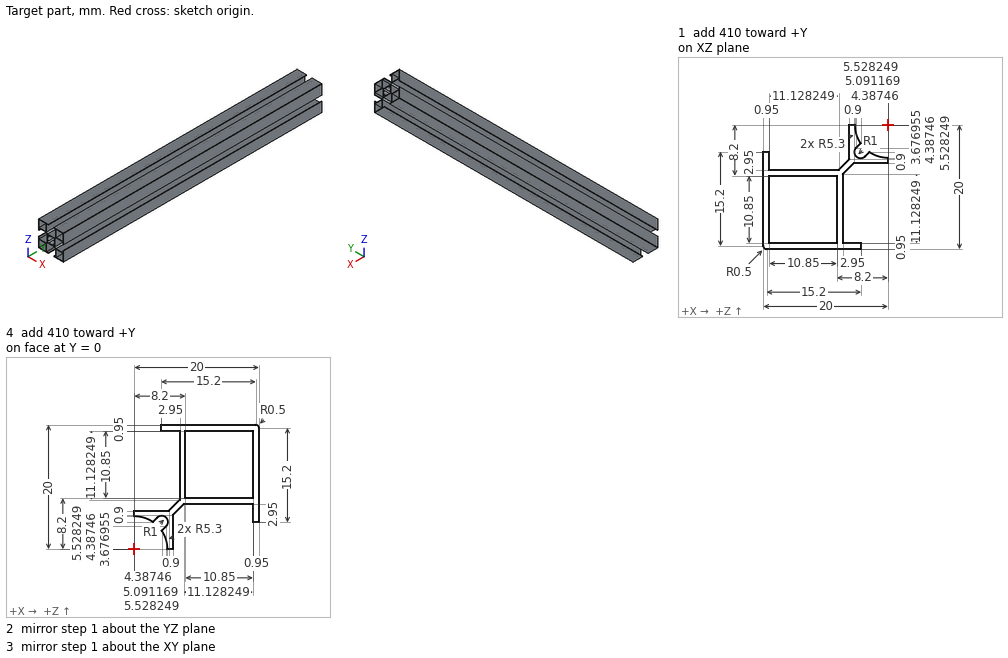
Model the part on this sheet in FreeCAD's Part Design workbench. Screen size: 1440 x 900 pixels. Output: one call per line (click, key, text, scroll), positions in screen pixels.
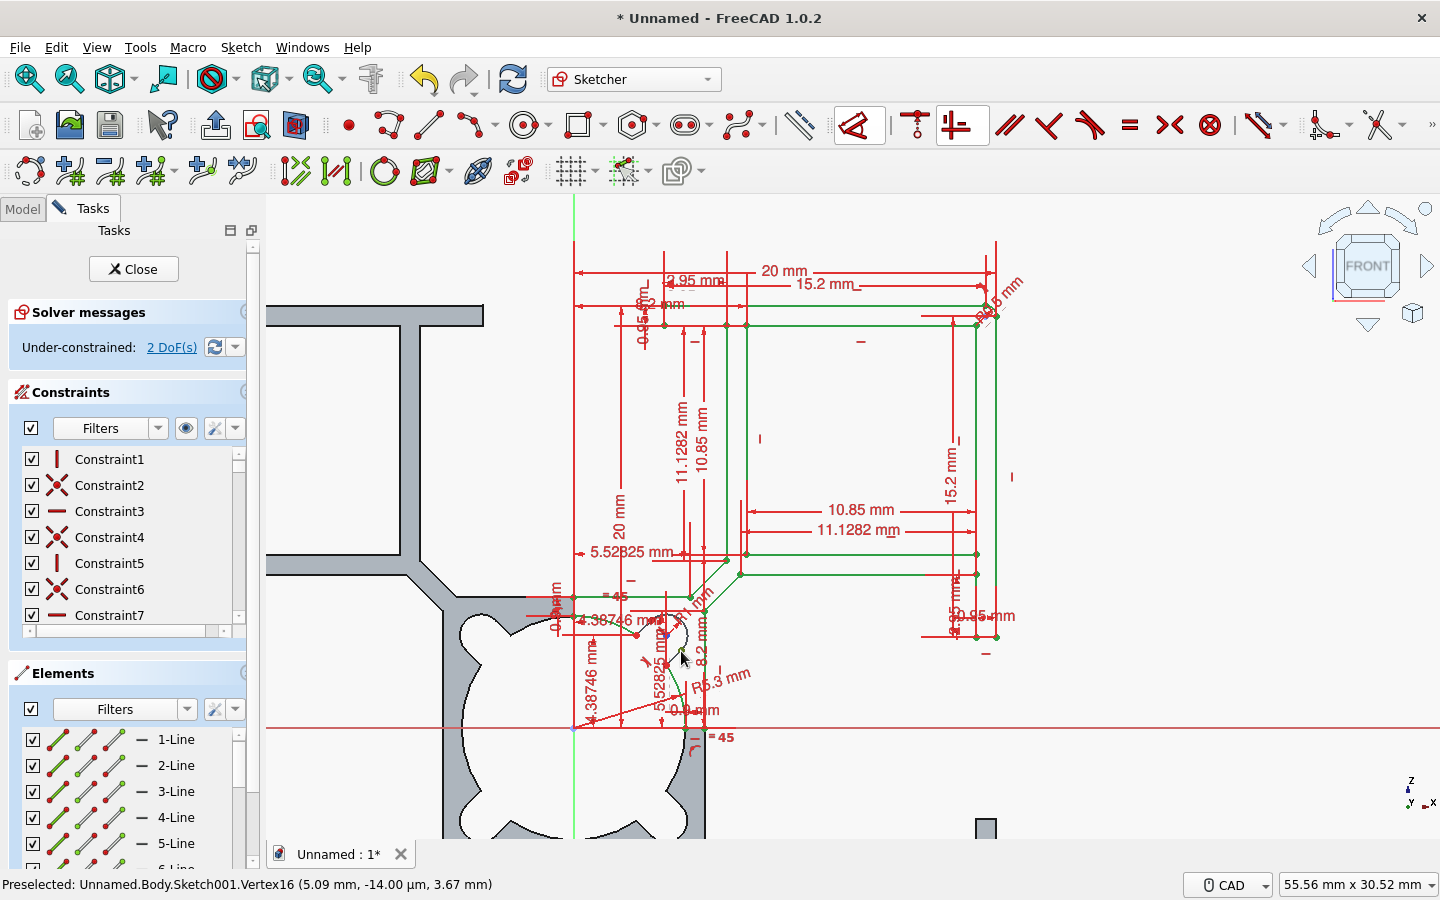
key(l)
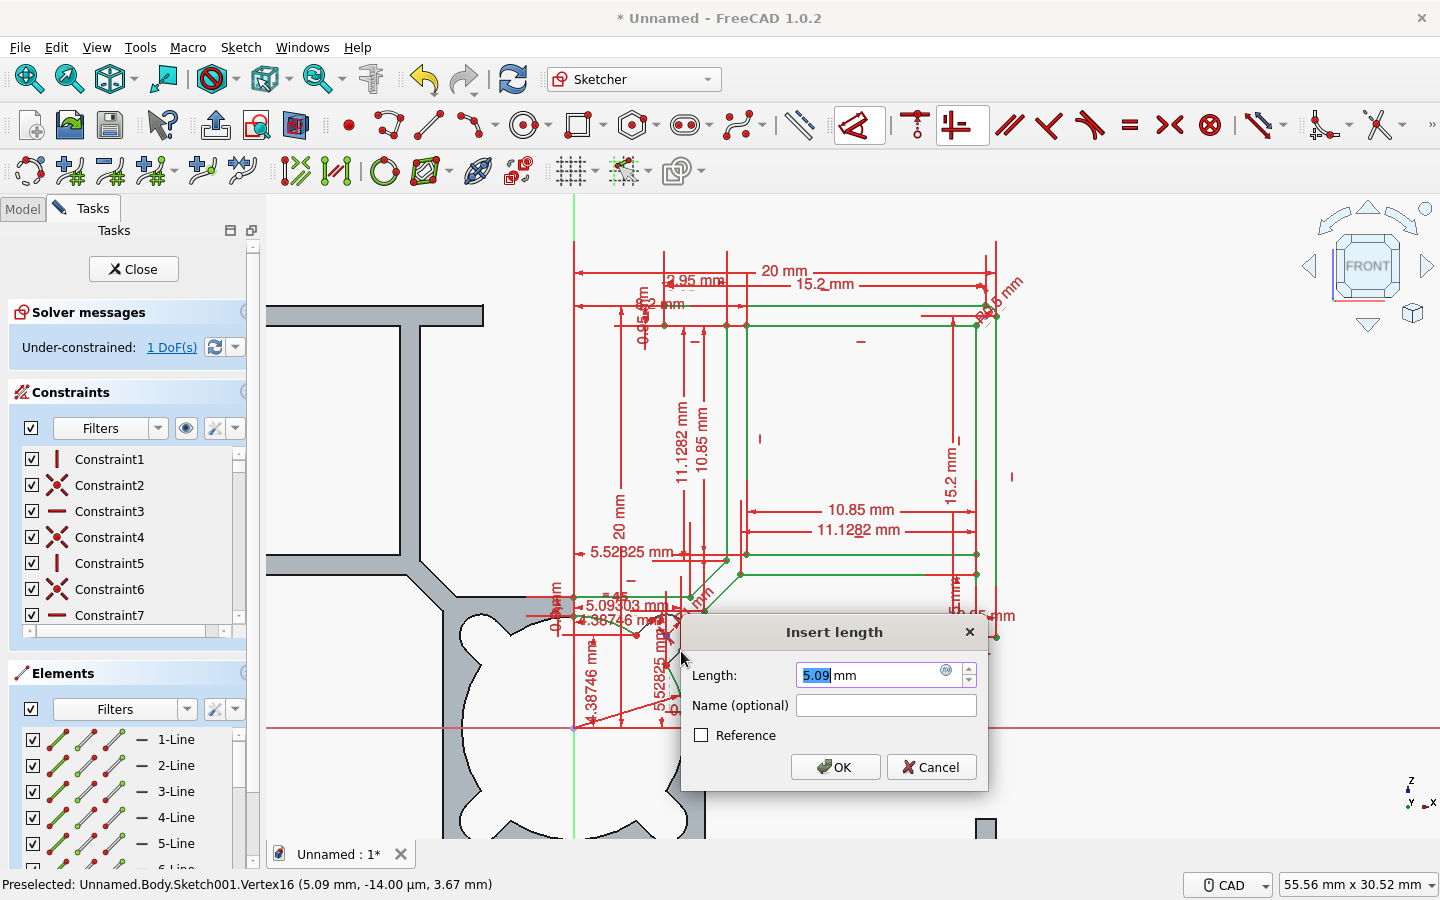
text(5.091169)
key(Return)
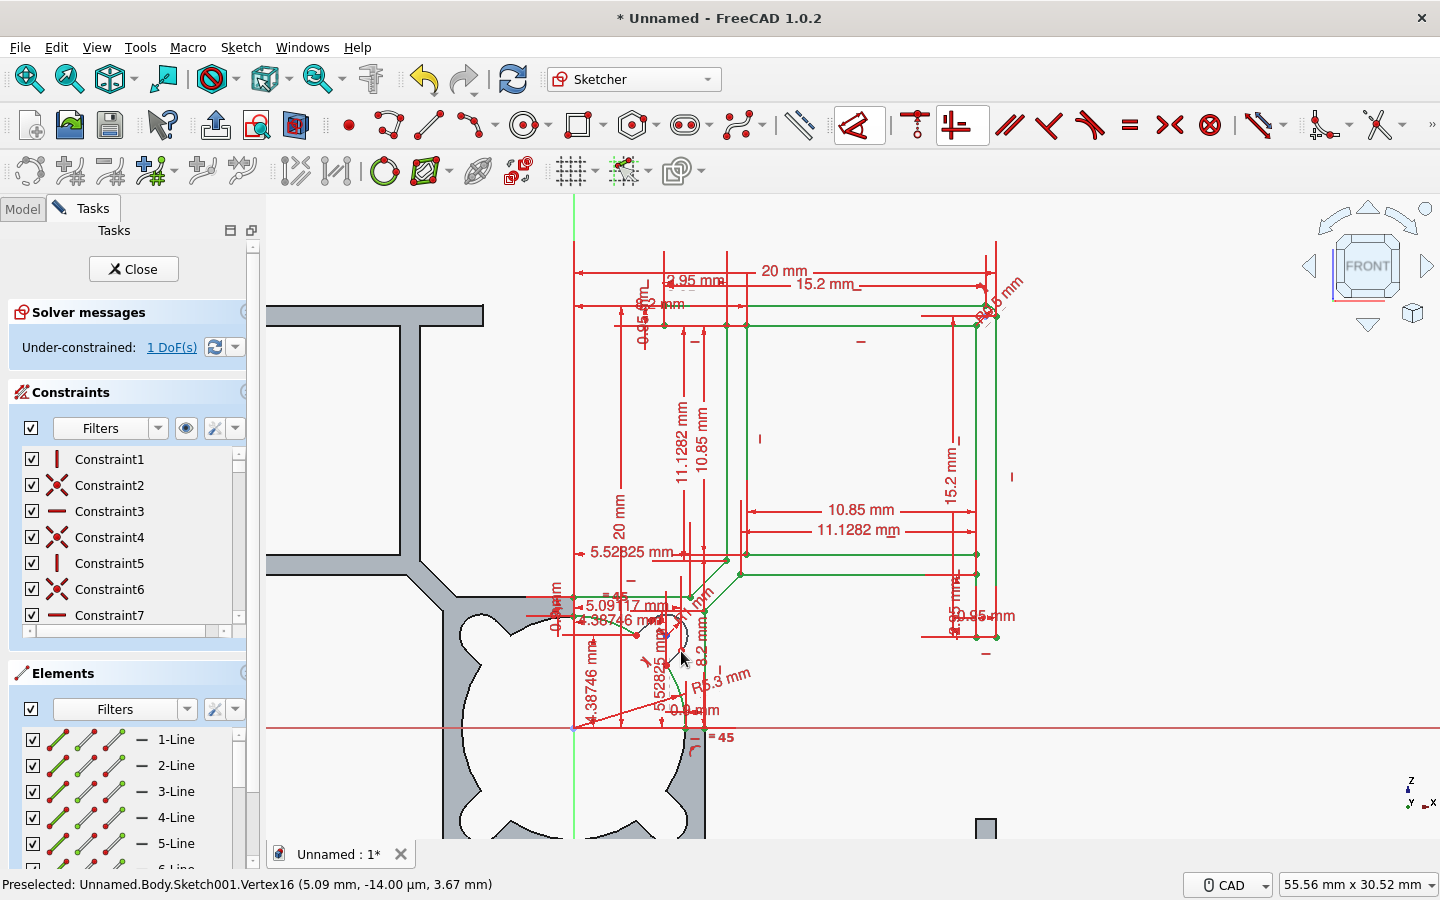
click(681, 651)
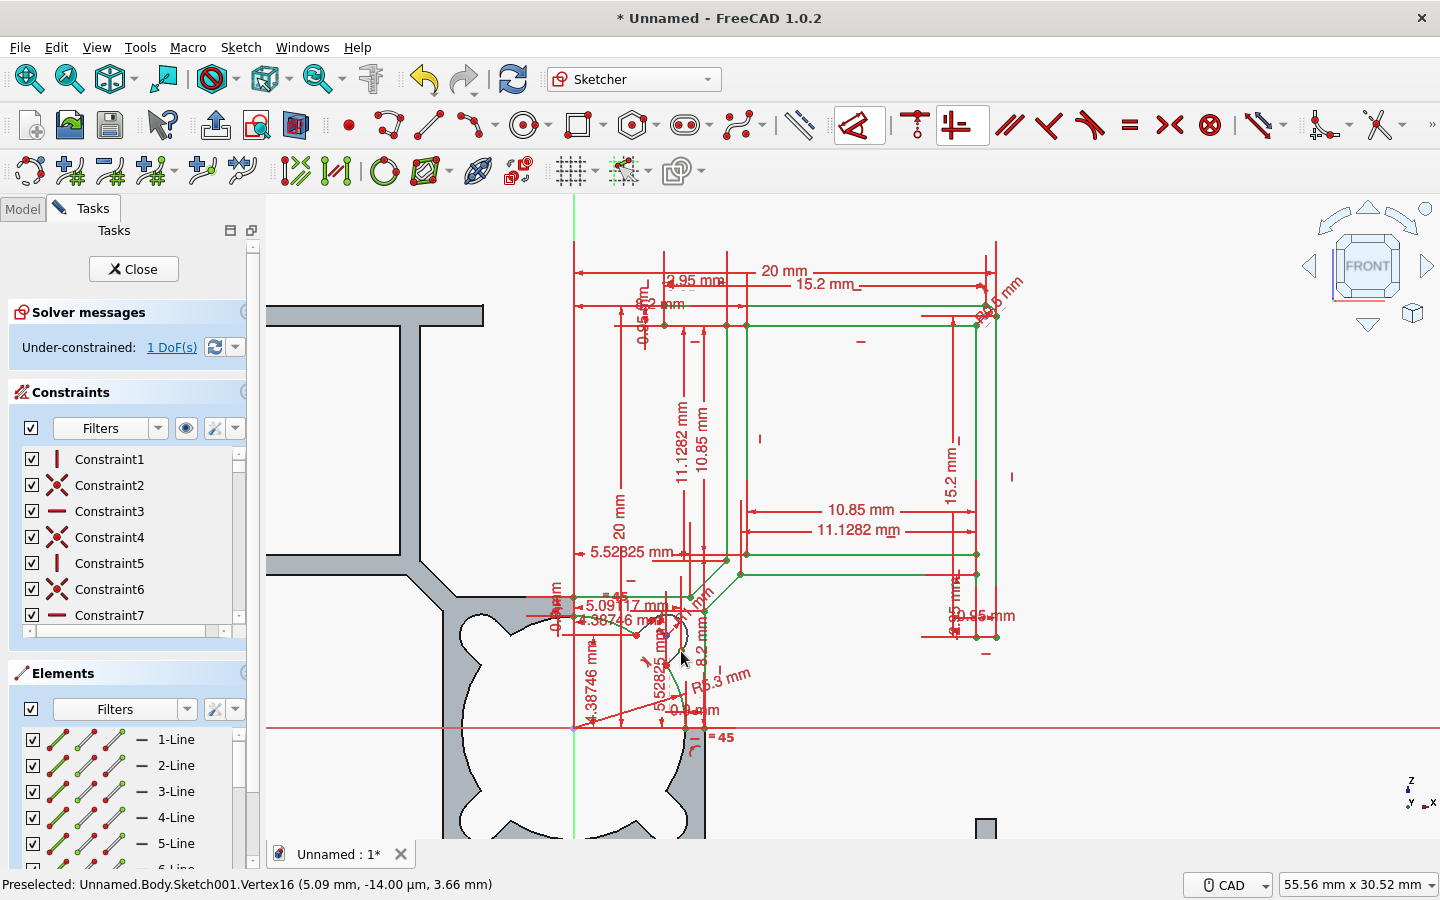
click(880, 126)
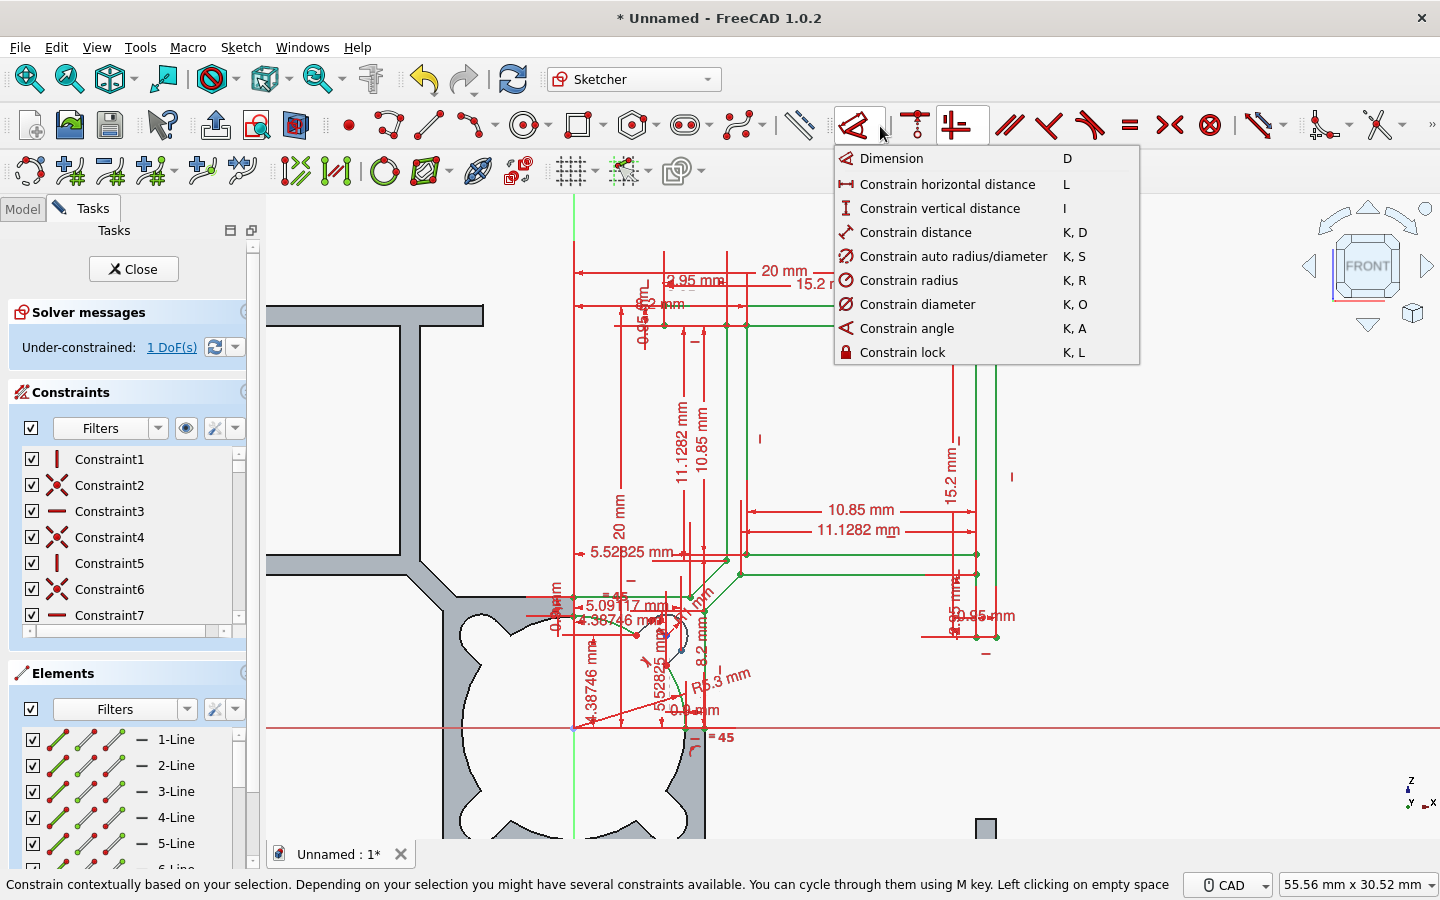
click(987, 208)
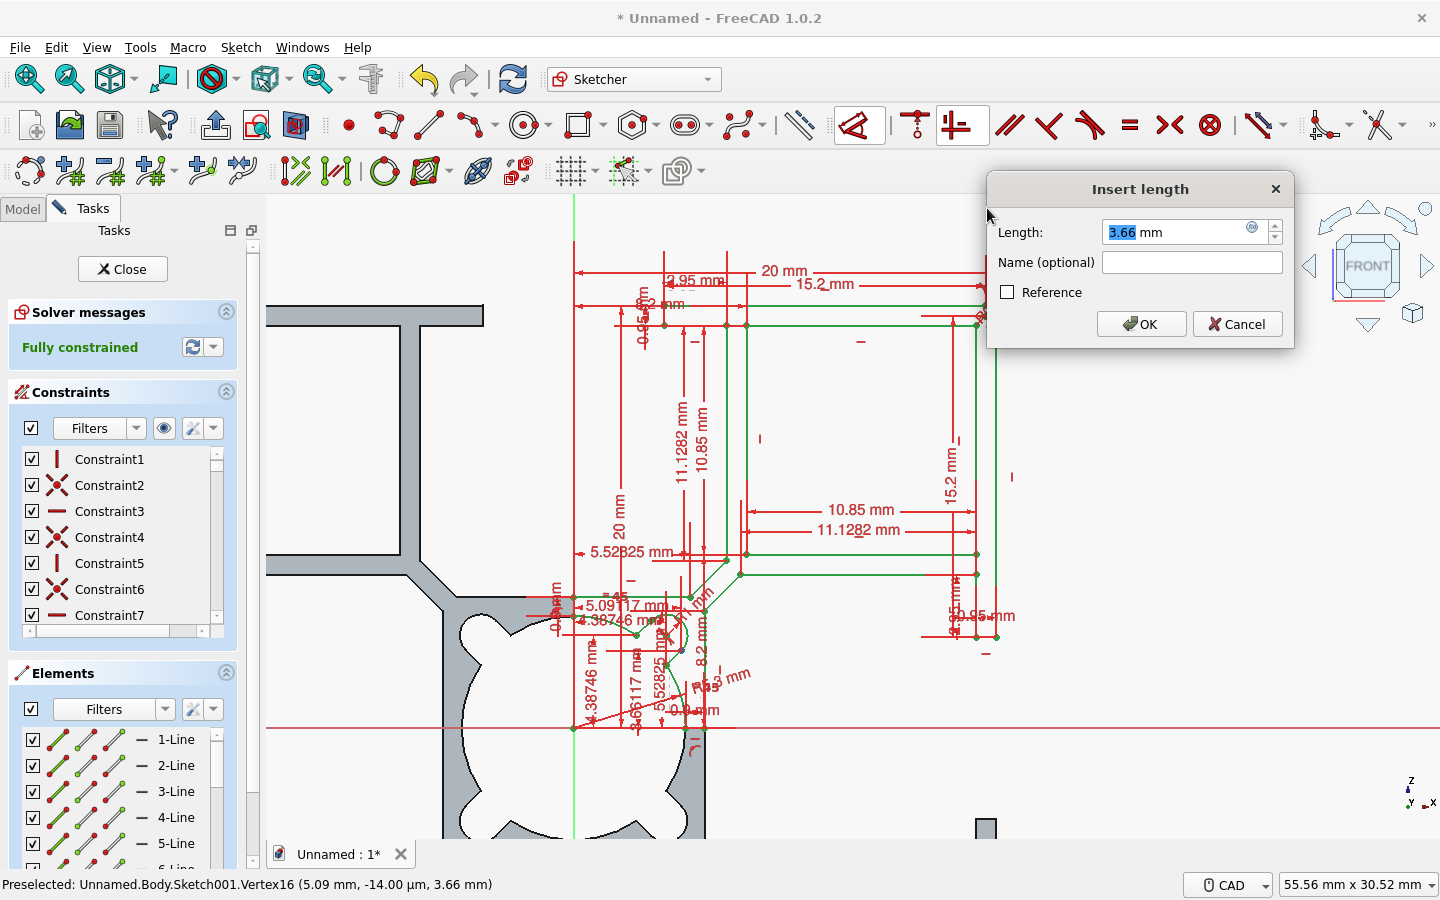
text(3.676955)
key(Return)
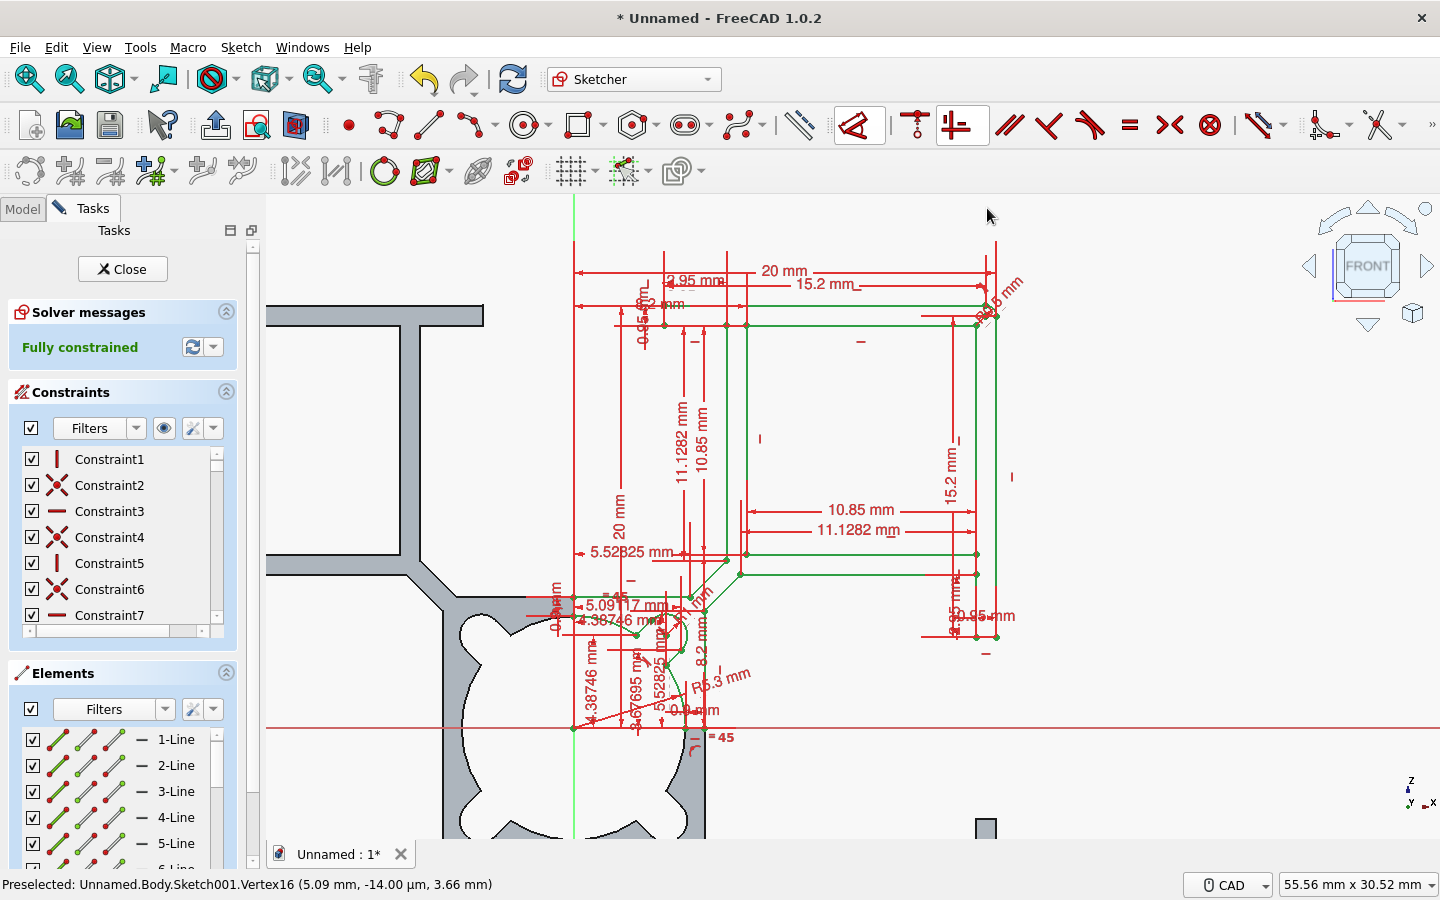
click(123, 269)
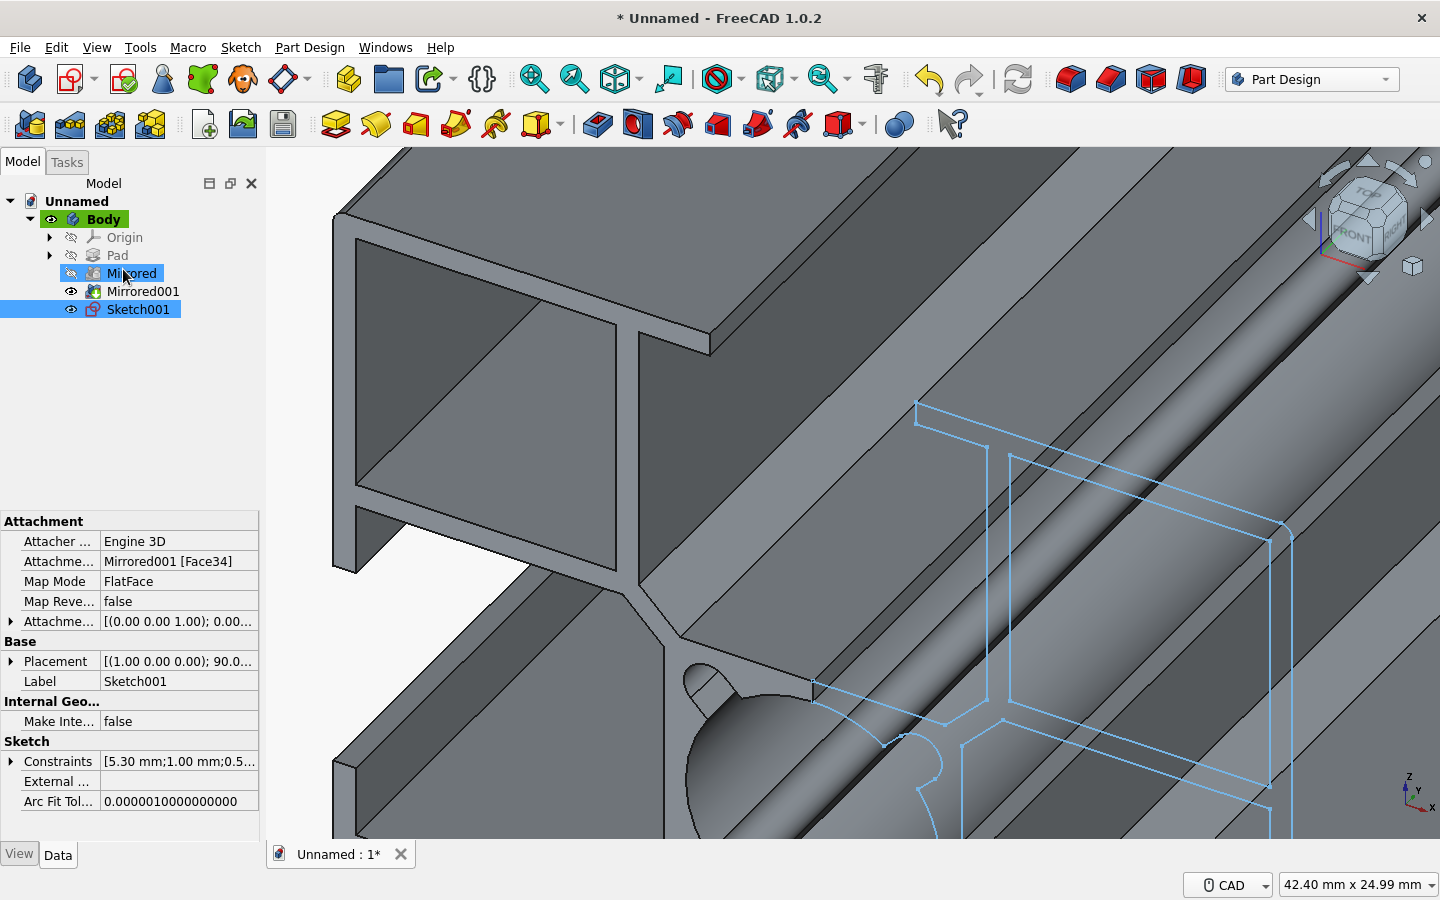
click(336, 124)